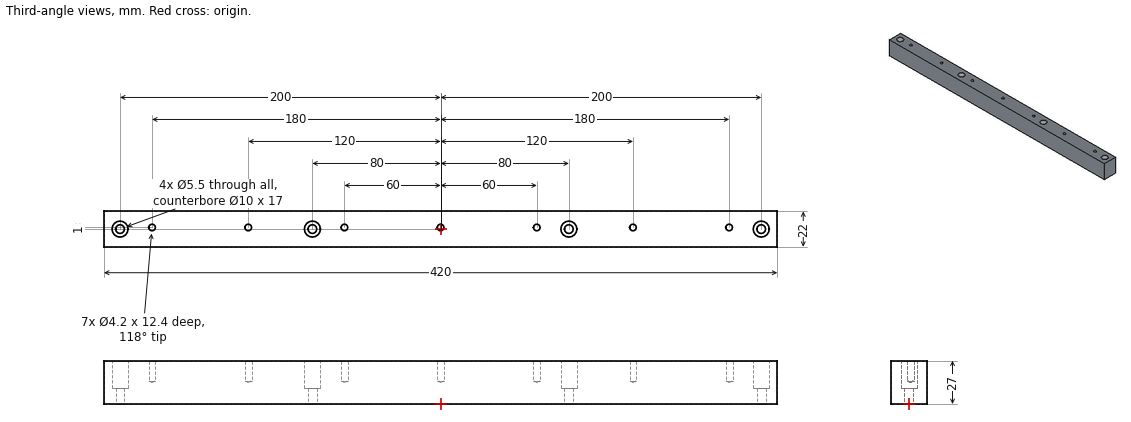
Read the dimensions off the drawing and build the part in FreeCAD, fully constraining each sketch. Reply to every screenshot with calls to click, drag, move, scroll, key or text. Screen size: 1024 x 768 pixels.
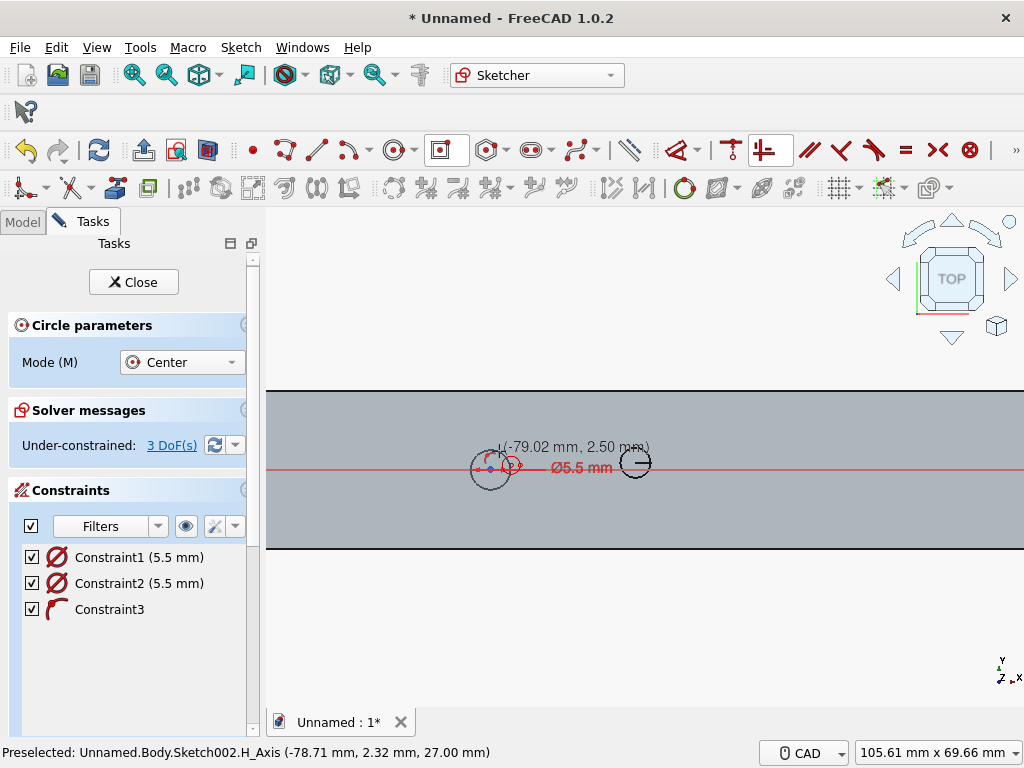
scroll(500, 455, down, 10)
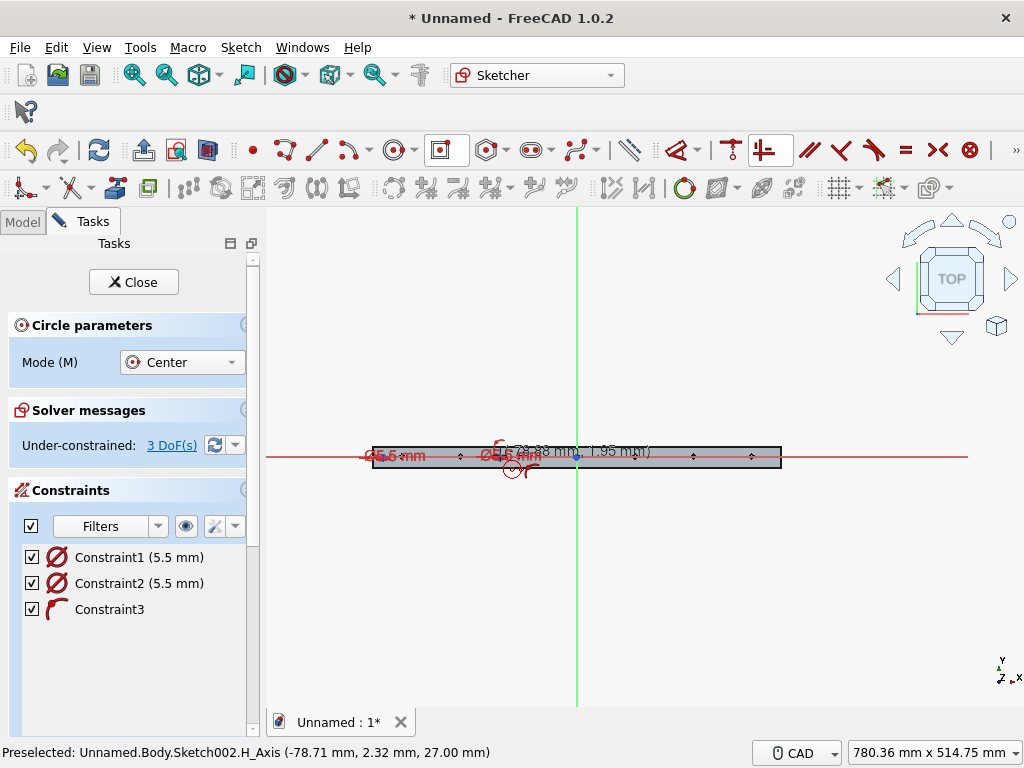
scroll(655, 457, up, 11)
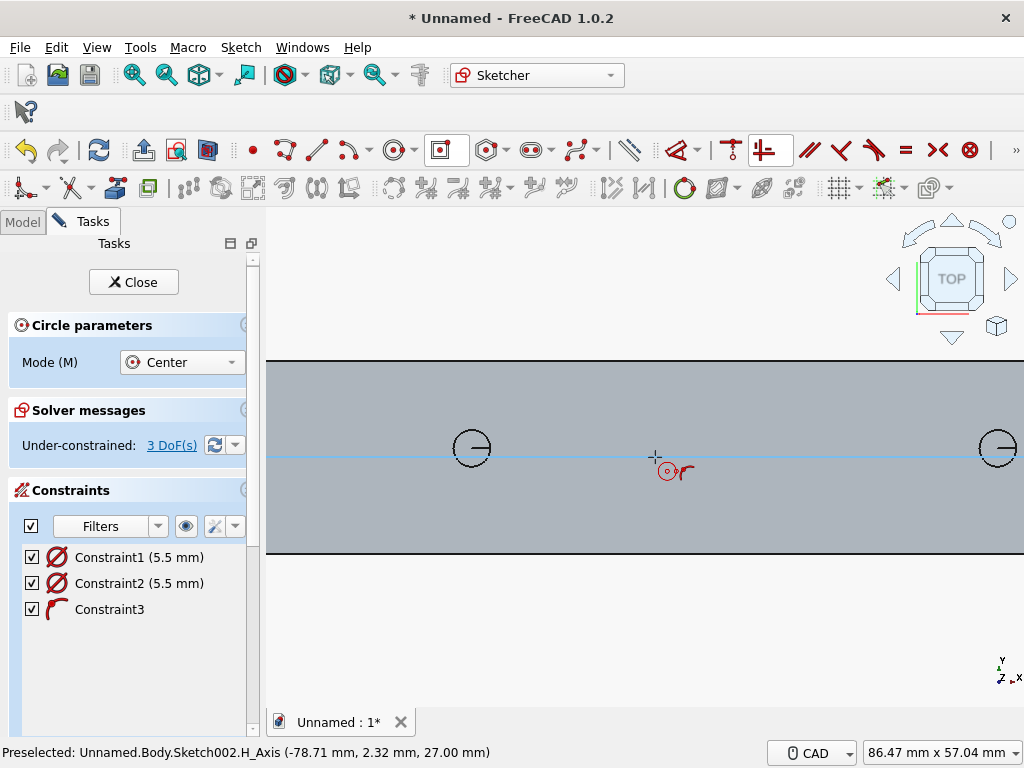
scroll(655, 457, down, 11)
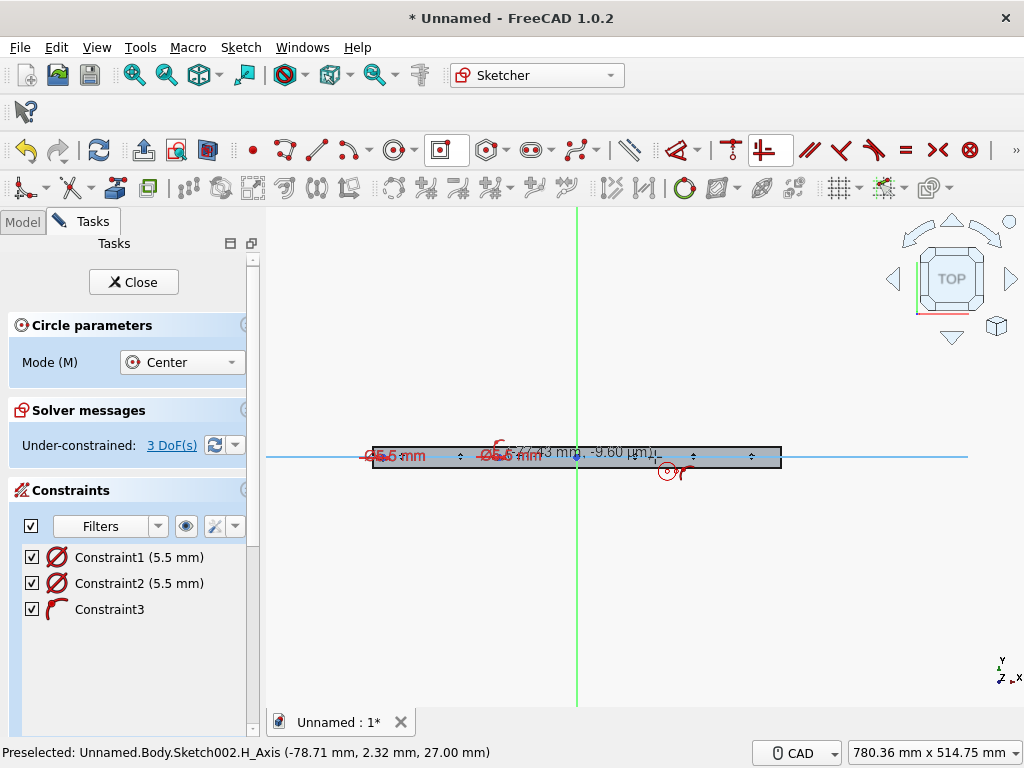
click(655, 457)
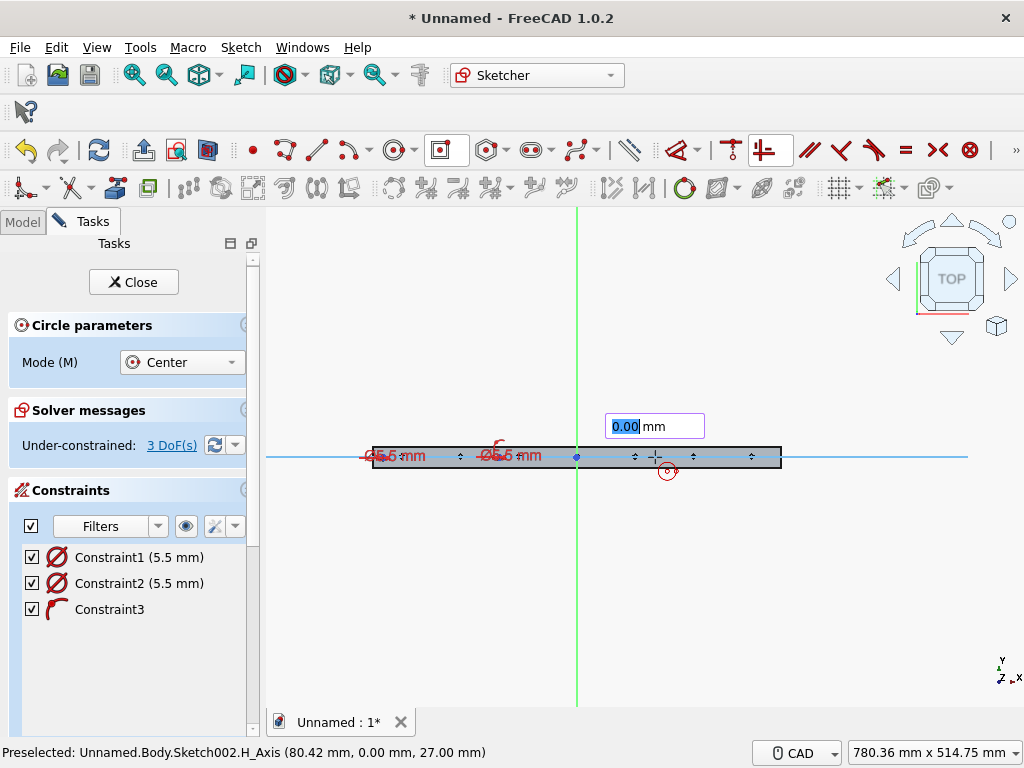
scroll(656, 455, up, 10)
move(649, 451)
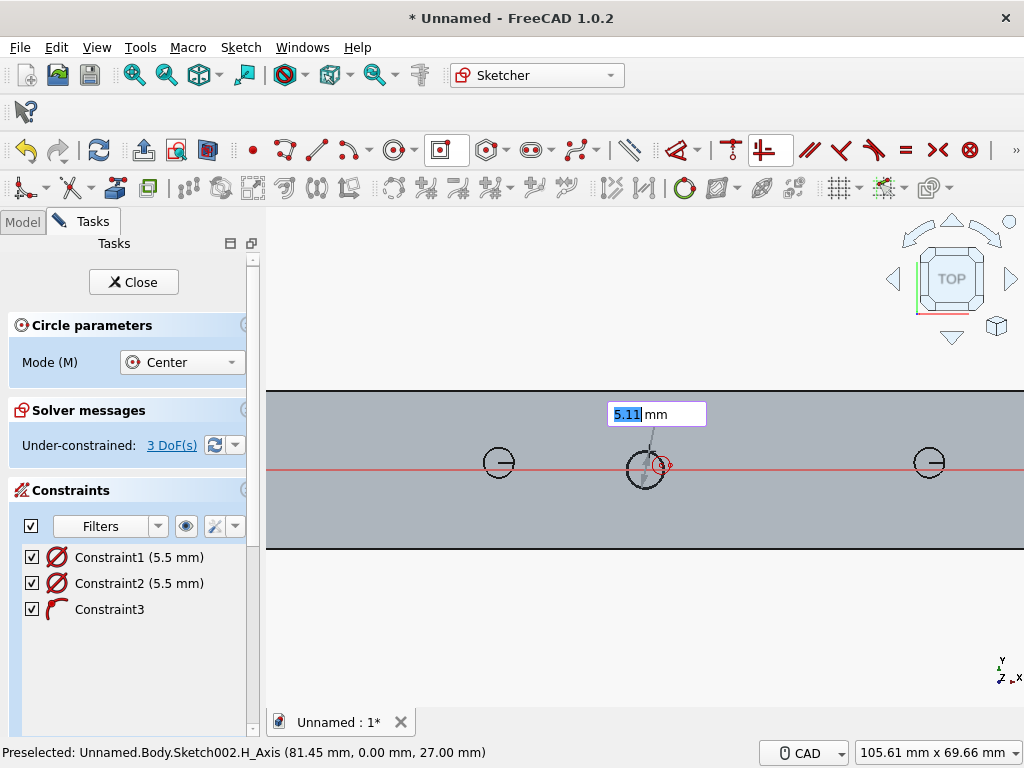
text(5.5)
key(Return)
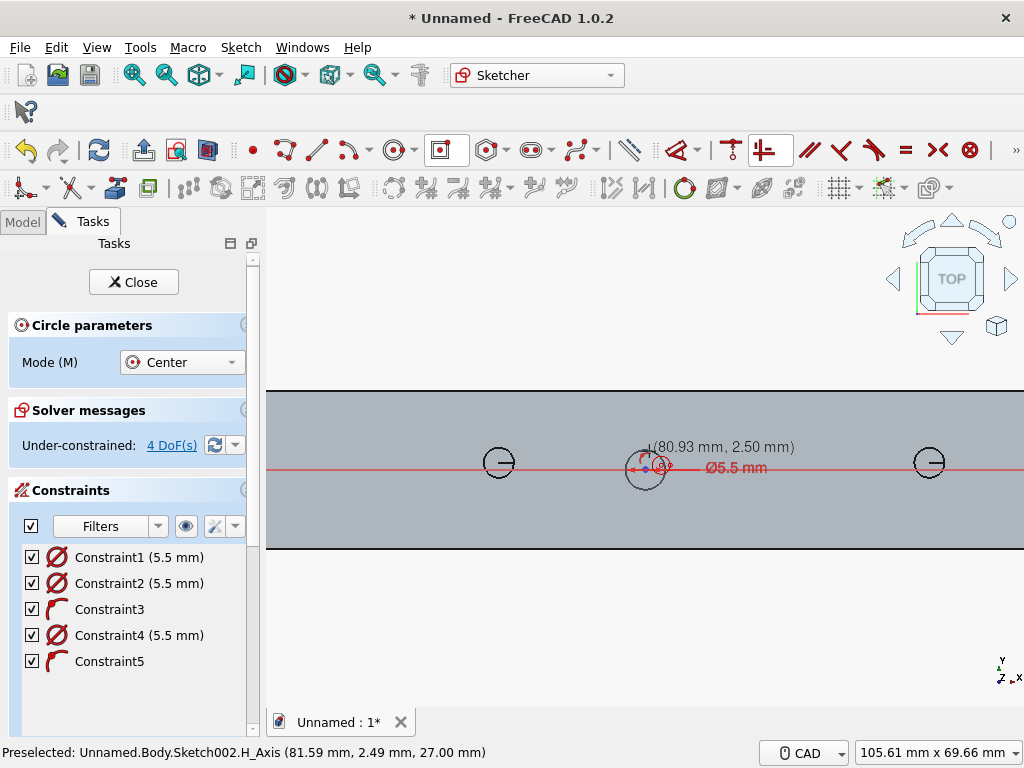
scroll(656, 455, down, 10)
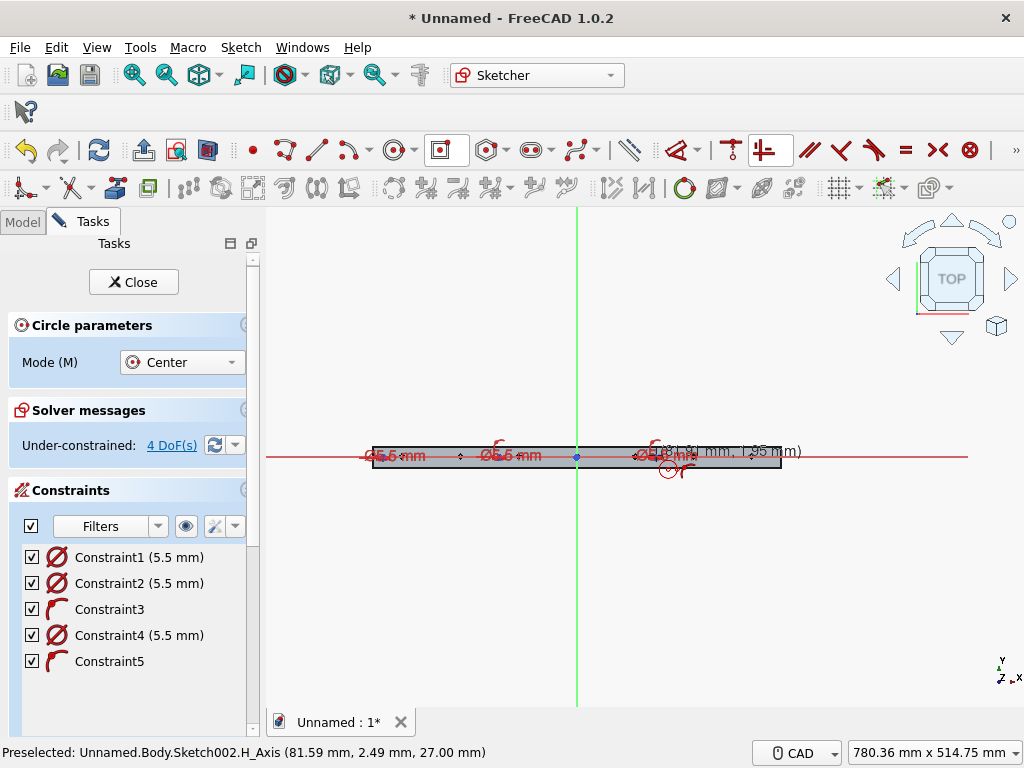
scroll(771, 457, up, 11)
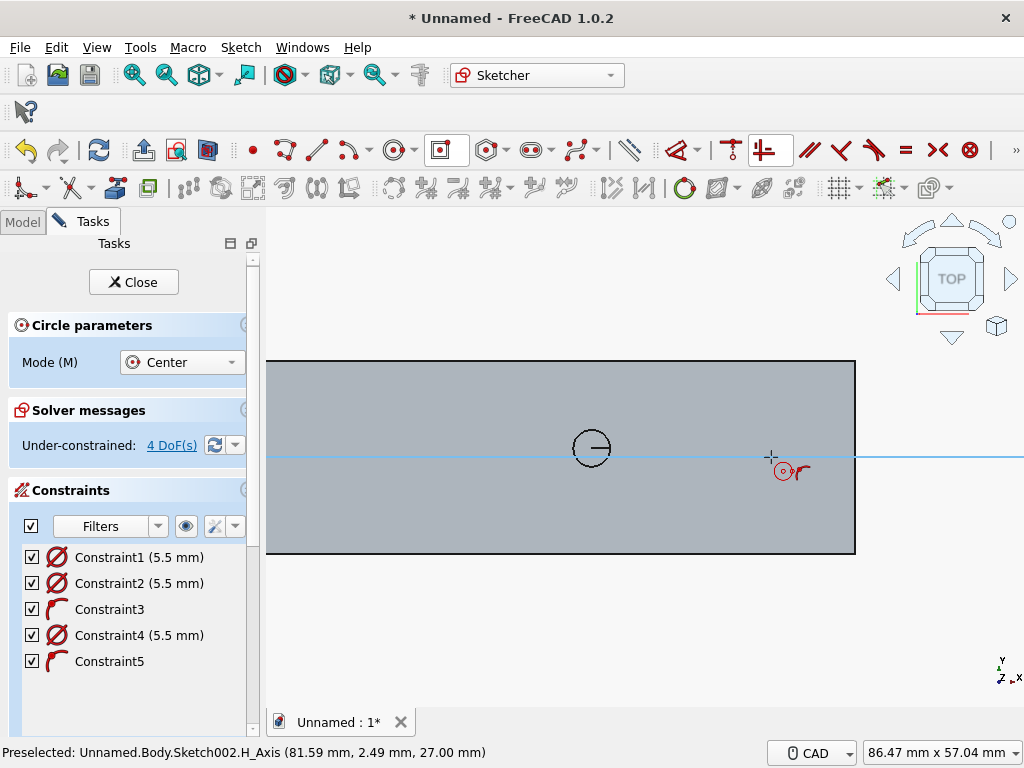
scroll(771, 457, down, 11)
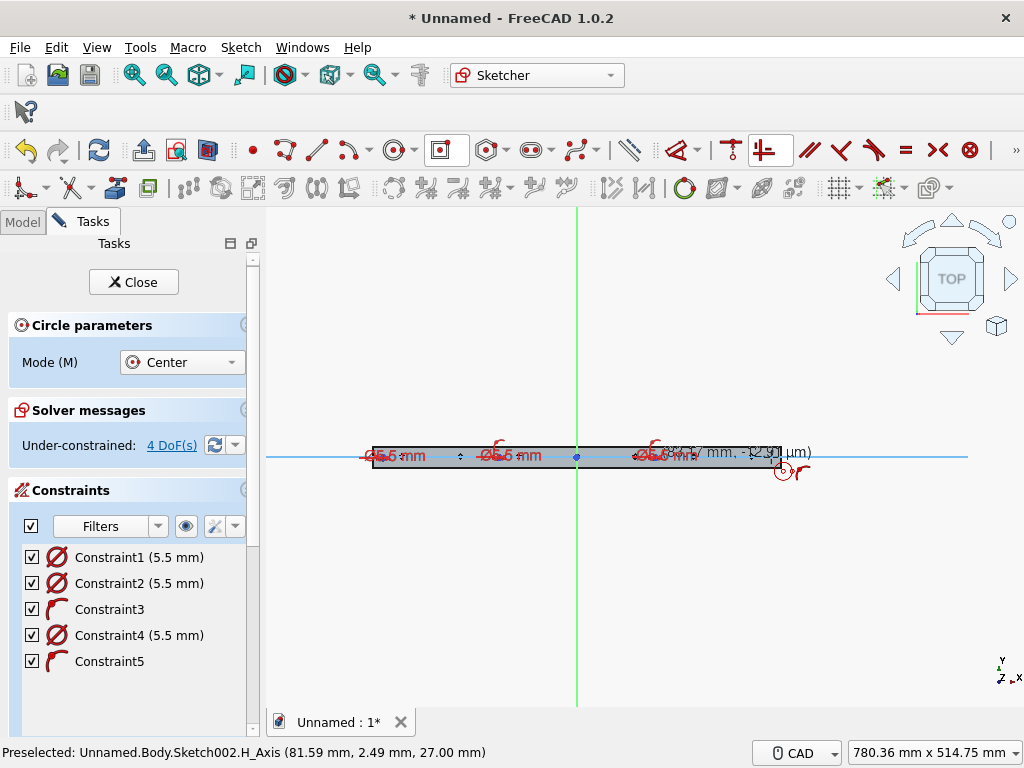
click(771, 457)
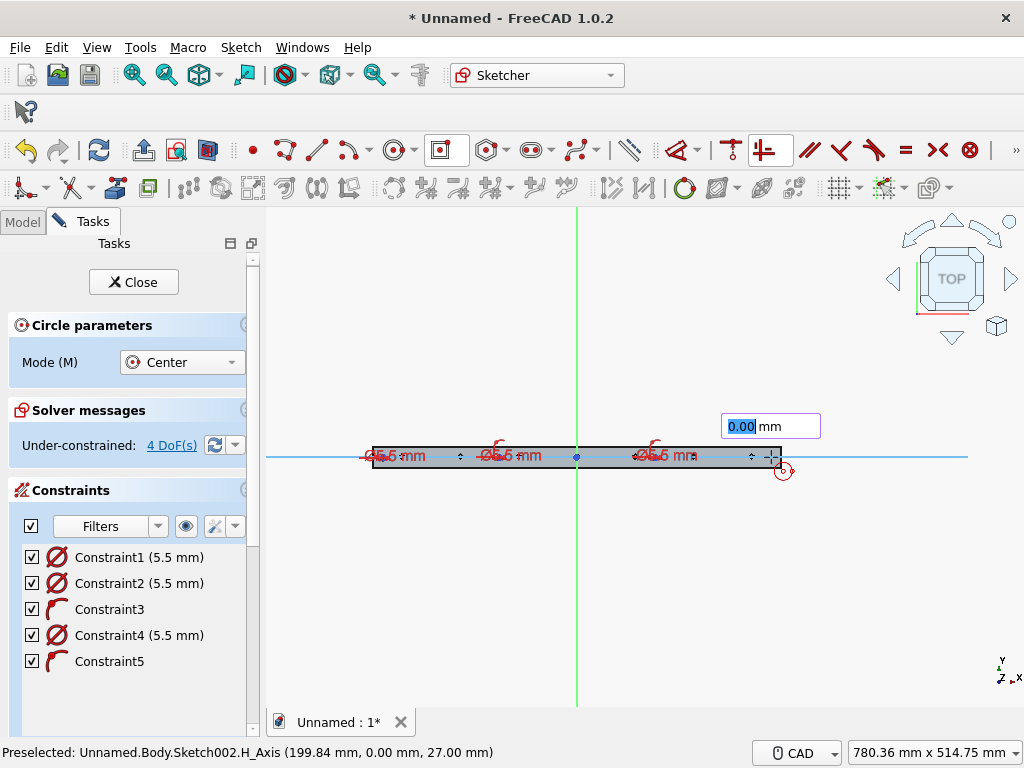
scroll(772, 455, up, 10)
move(768, 451)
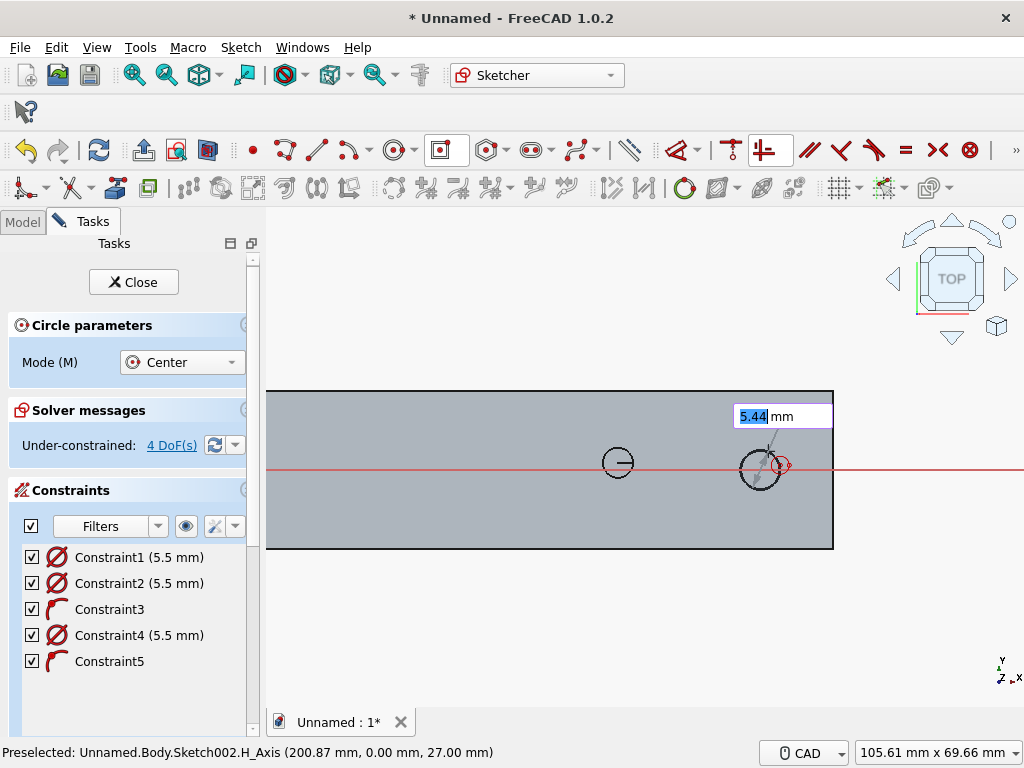
text(5.5)
key(Return)
key(Escape)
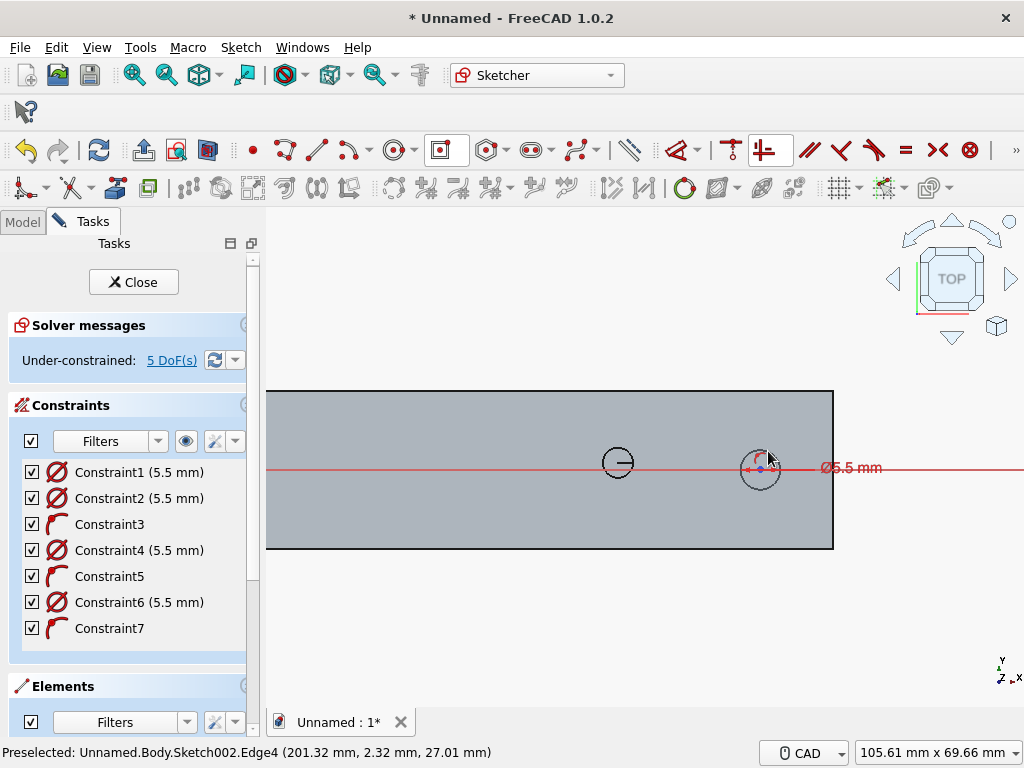
scroll(772, 455, down, 10)